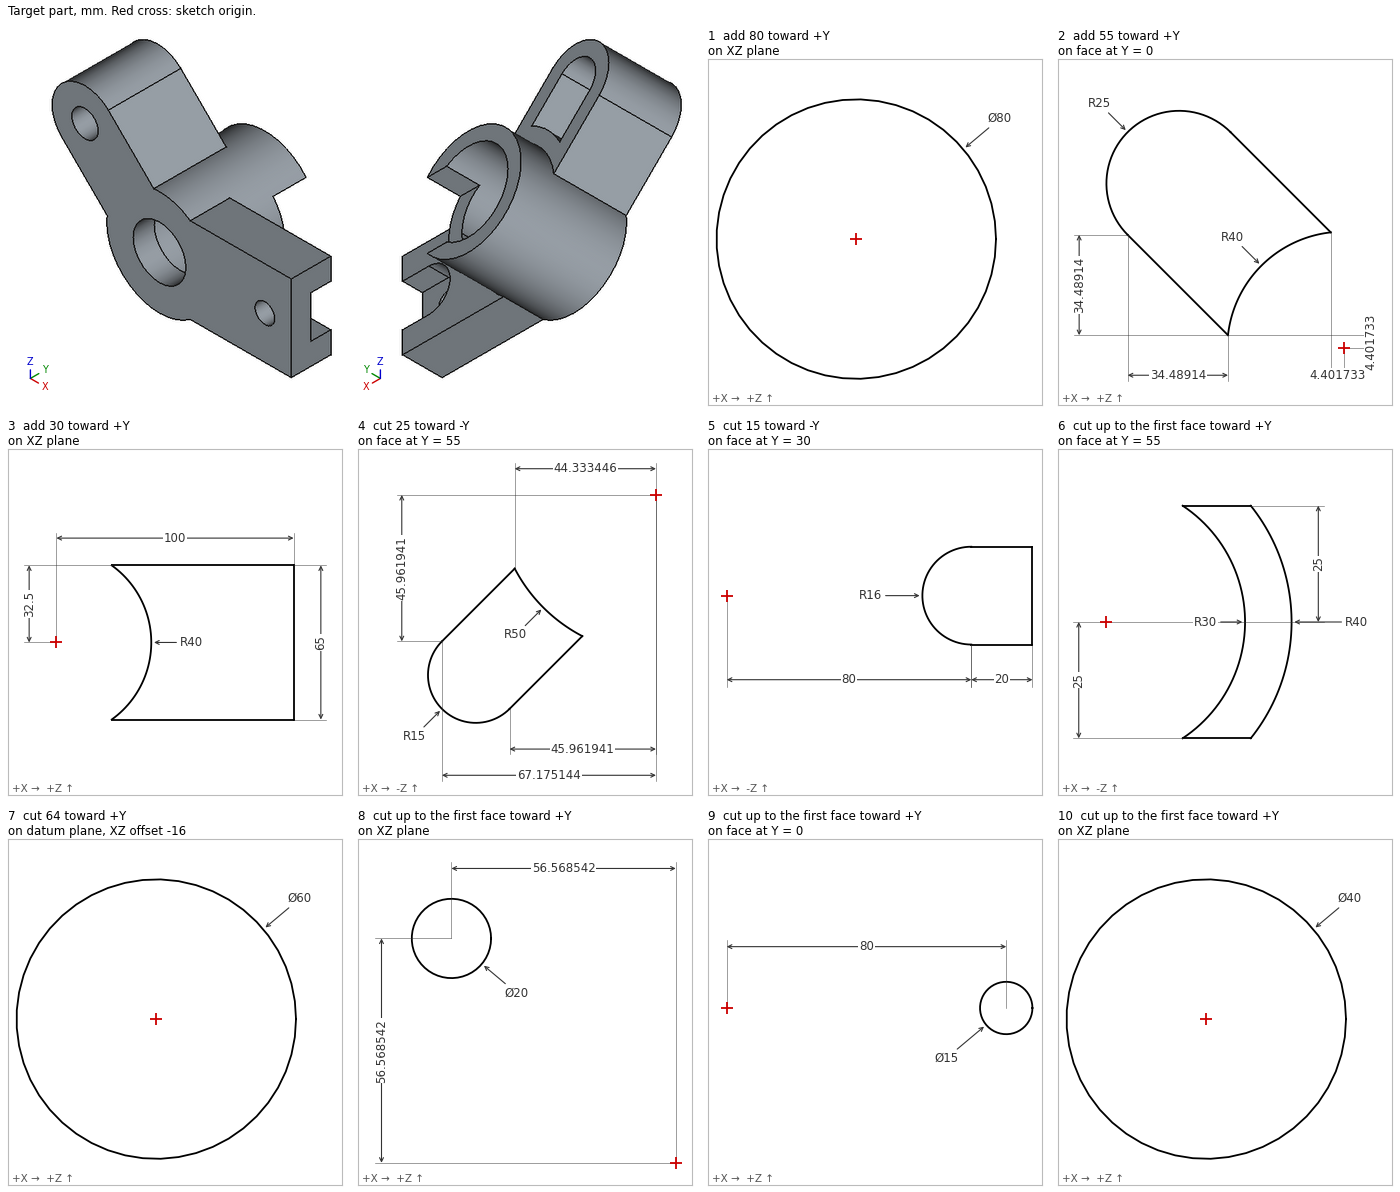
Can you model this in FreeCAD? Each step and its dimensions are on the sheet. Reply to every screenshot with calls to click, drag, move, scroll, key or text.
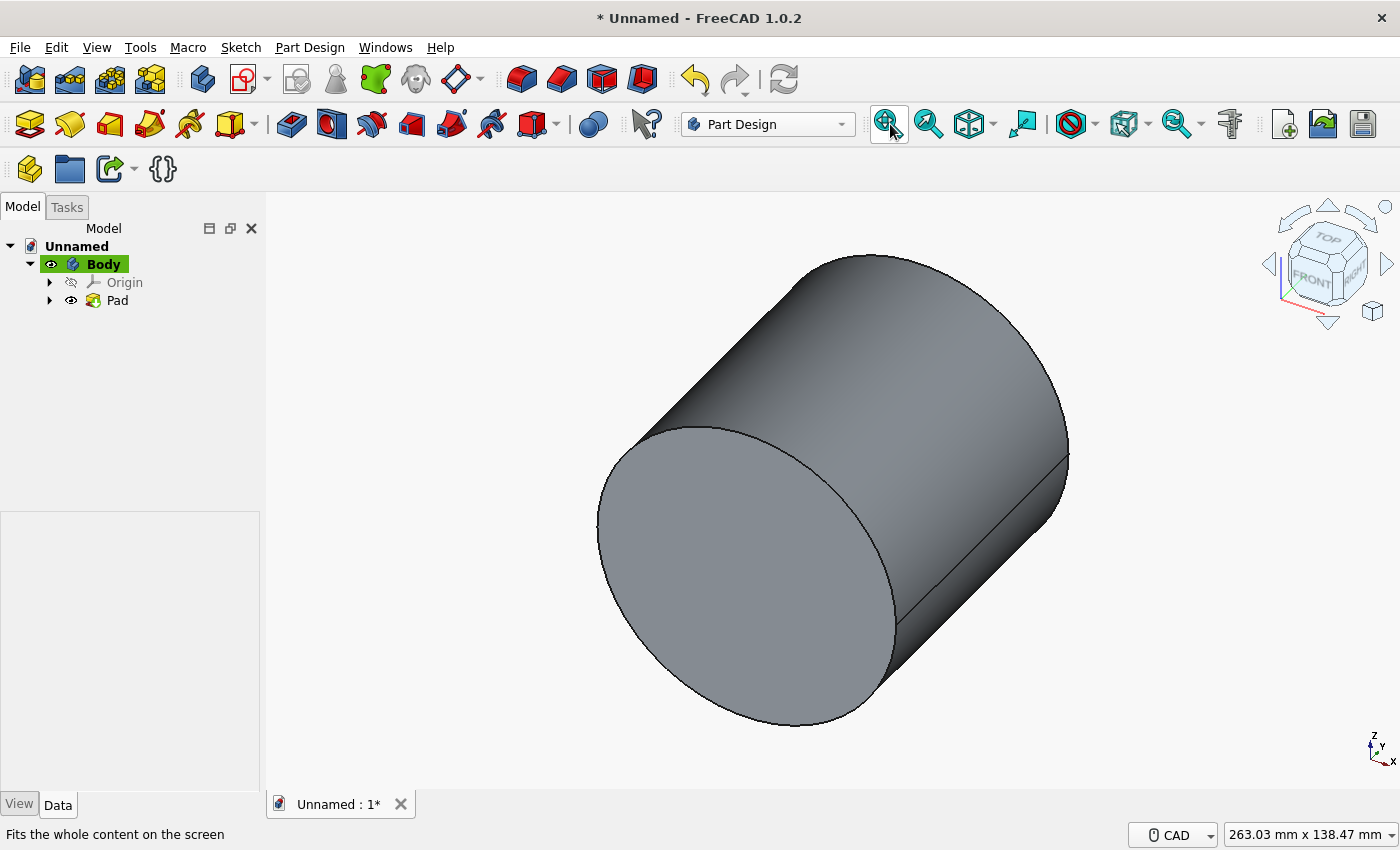
click(747, 575)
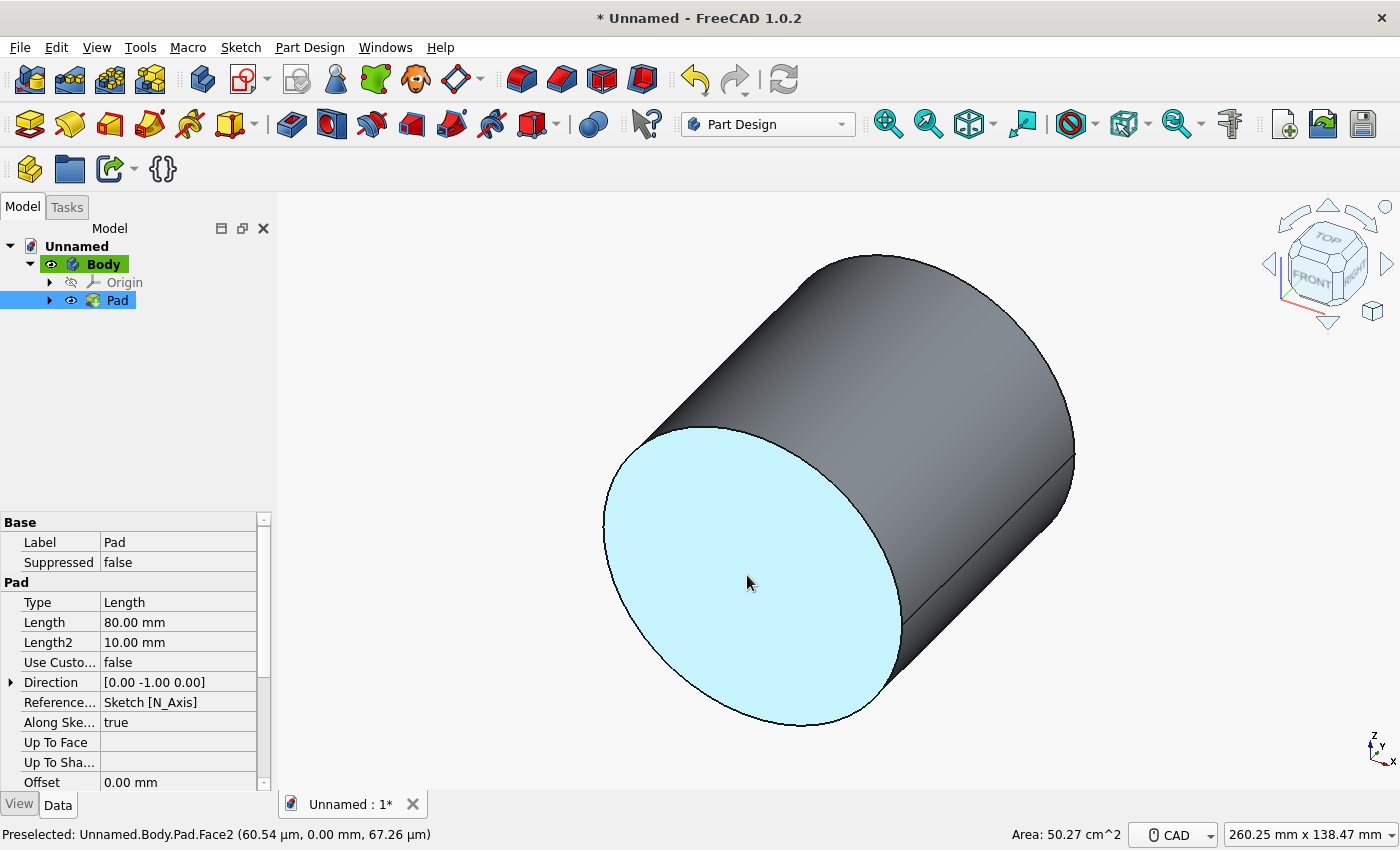
click(244, 80)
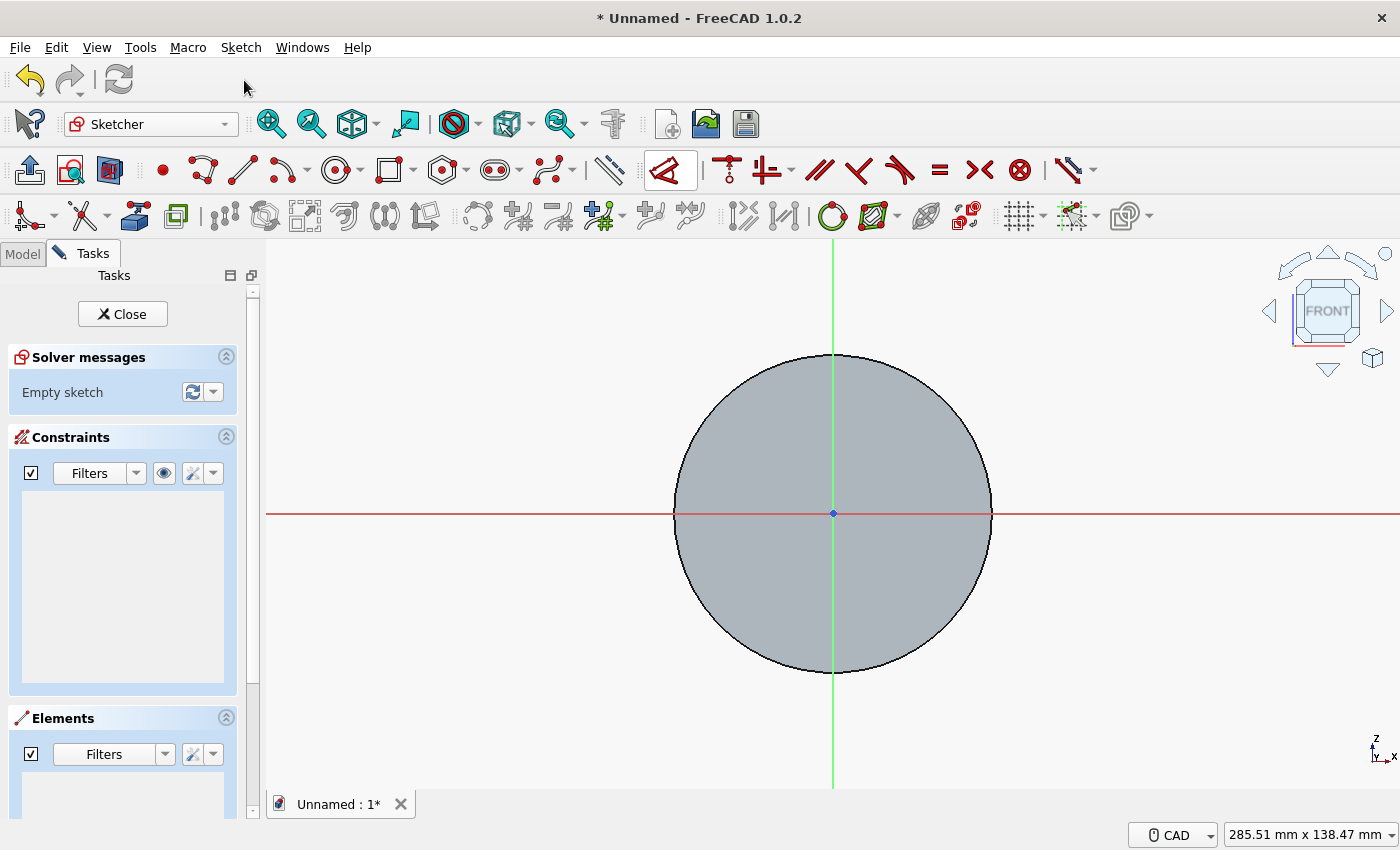
scroll(1121, 761, down, 1)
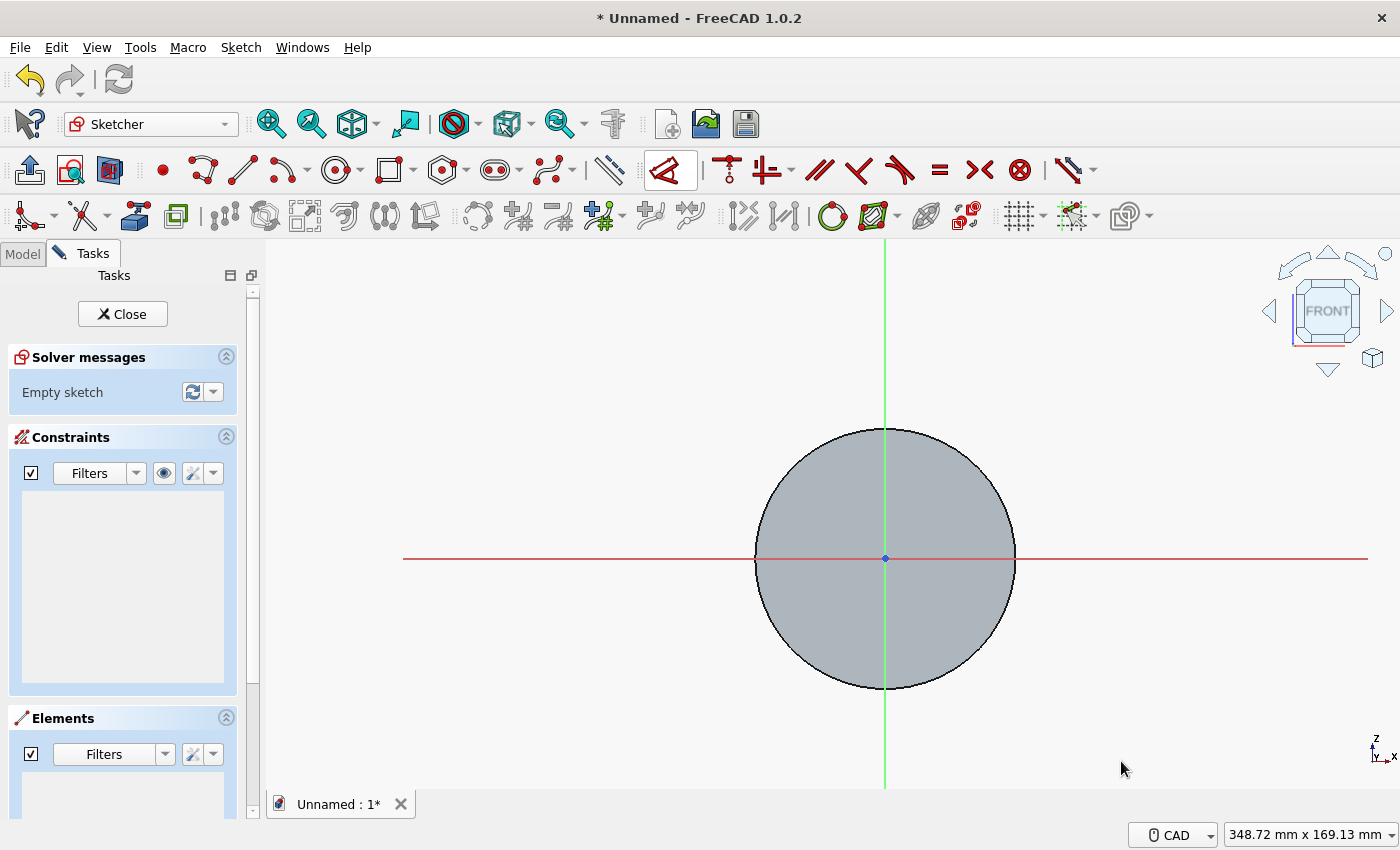
scroll(765, 284, up, 2)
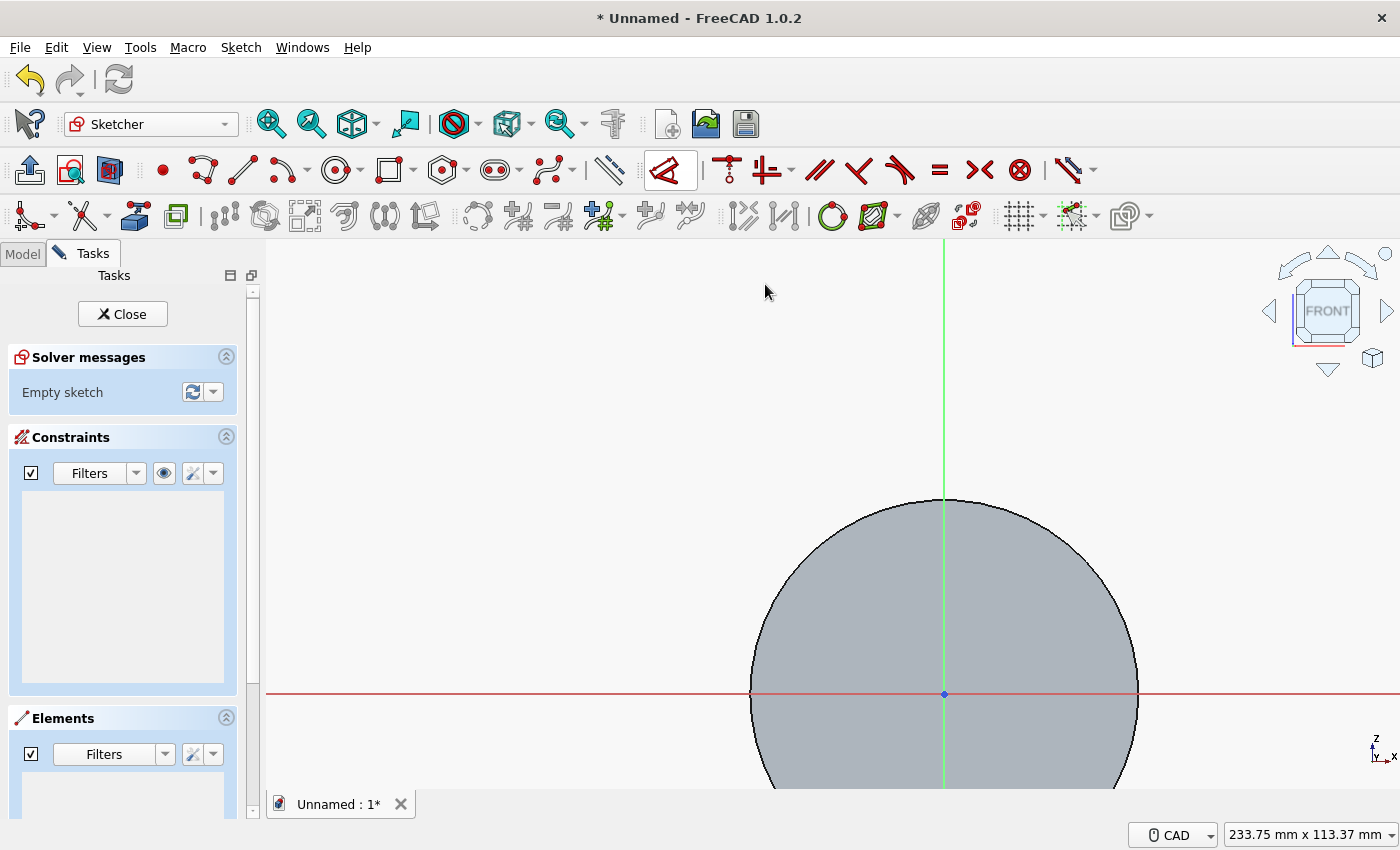
click(244, 170)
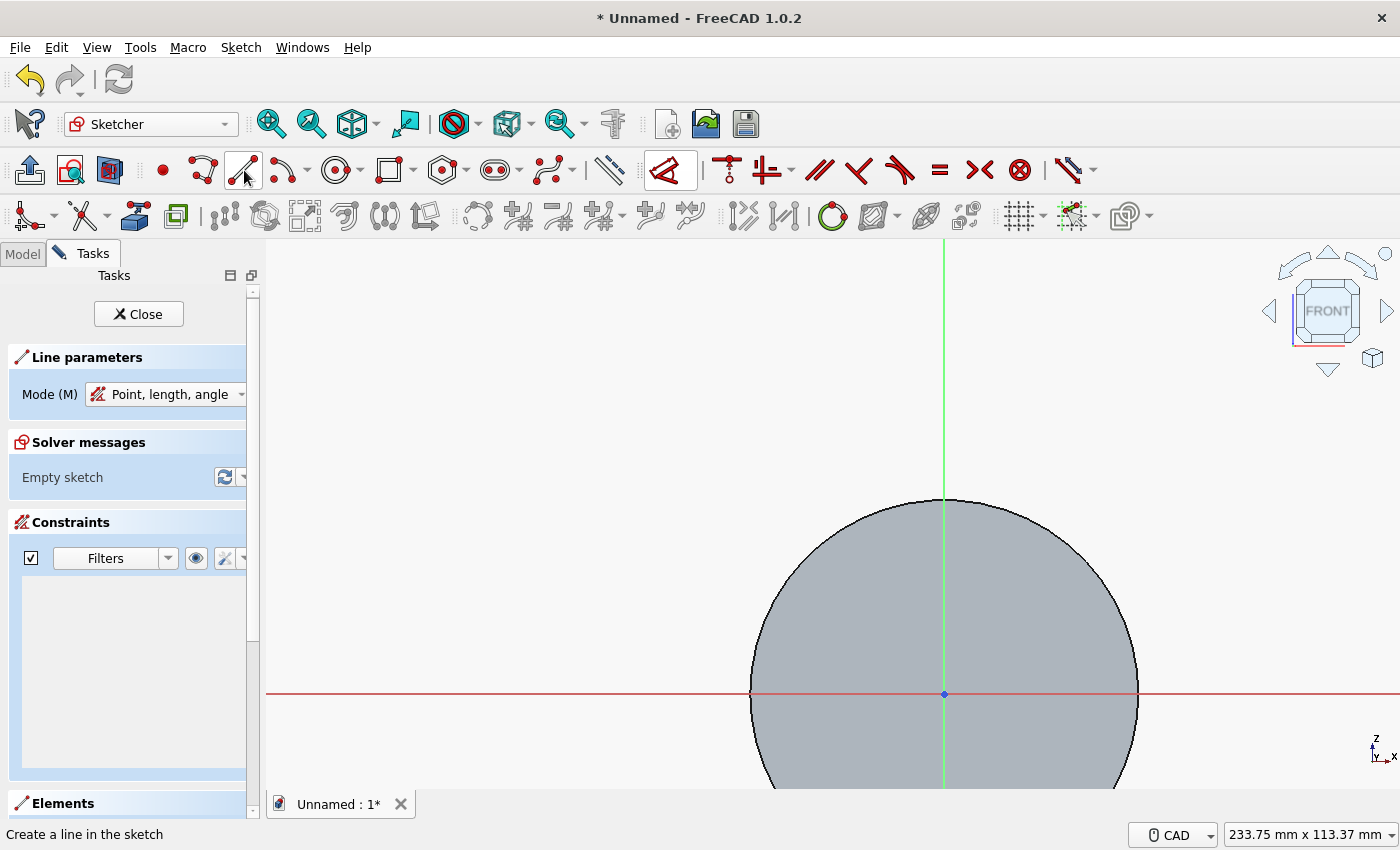
click(751, 673)
click(584, 505)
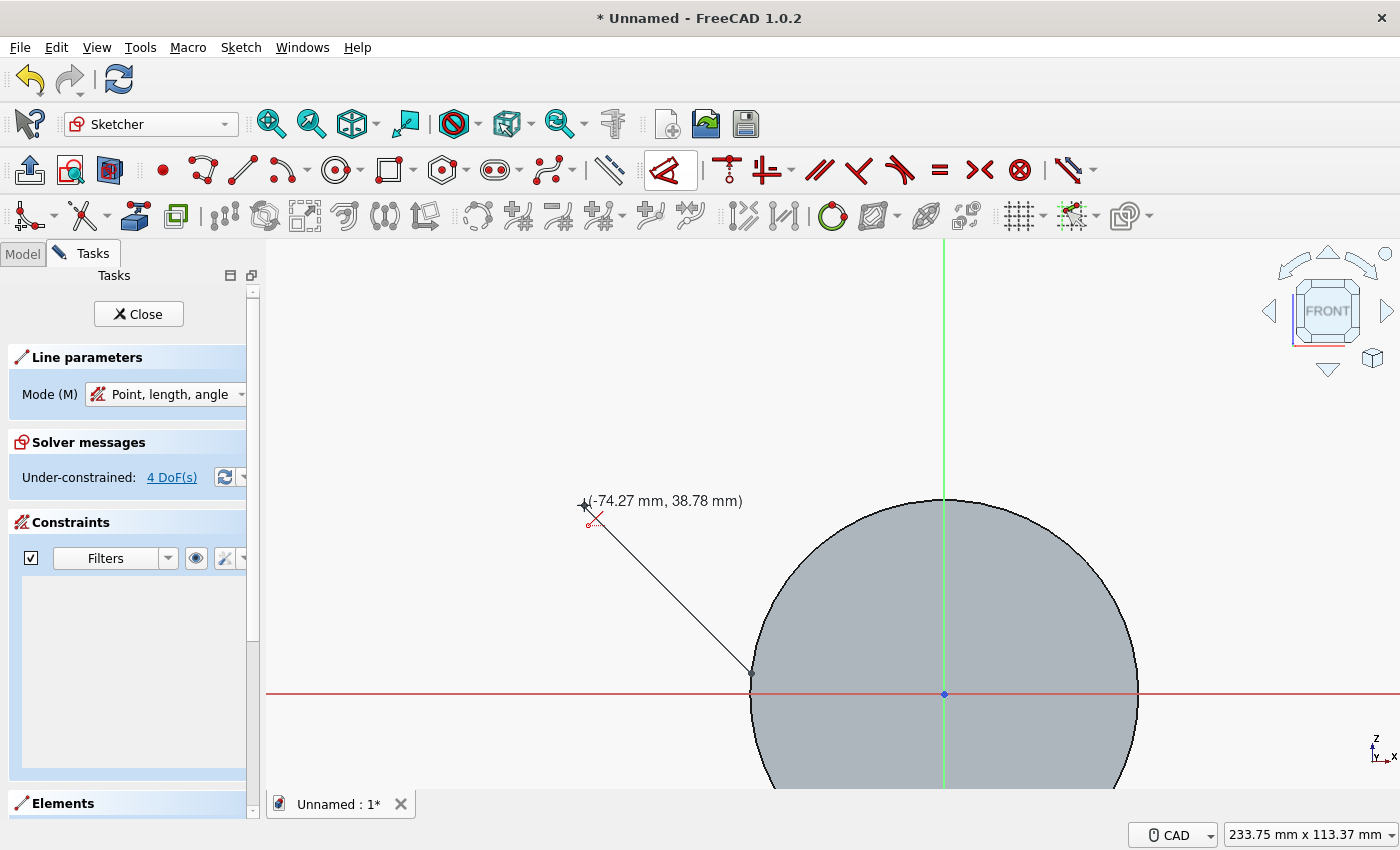
click(756, 334)
click(923, 501)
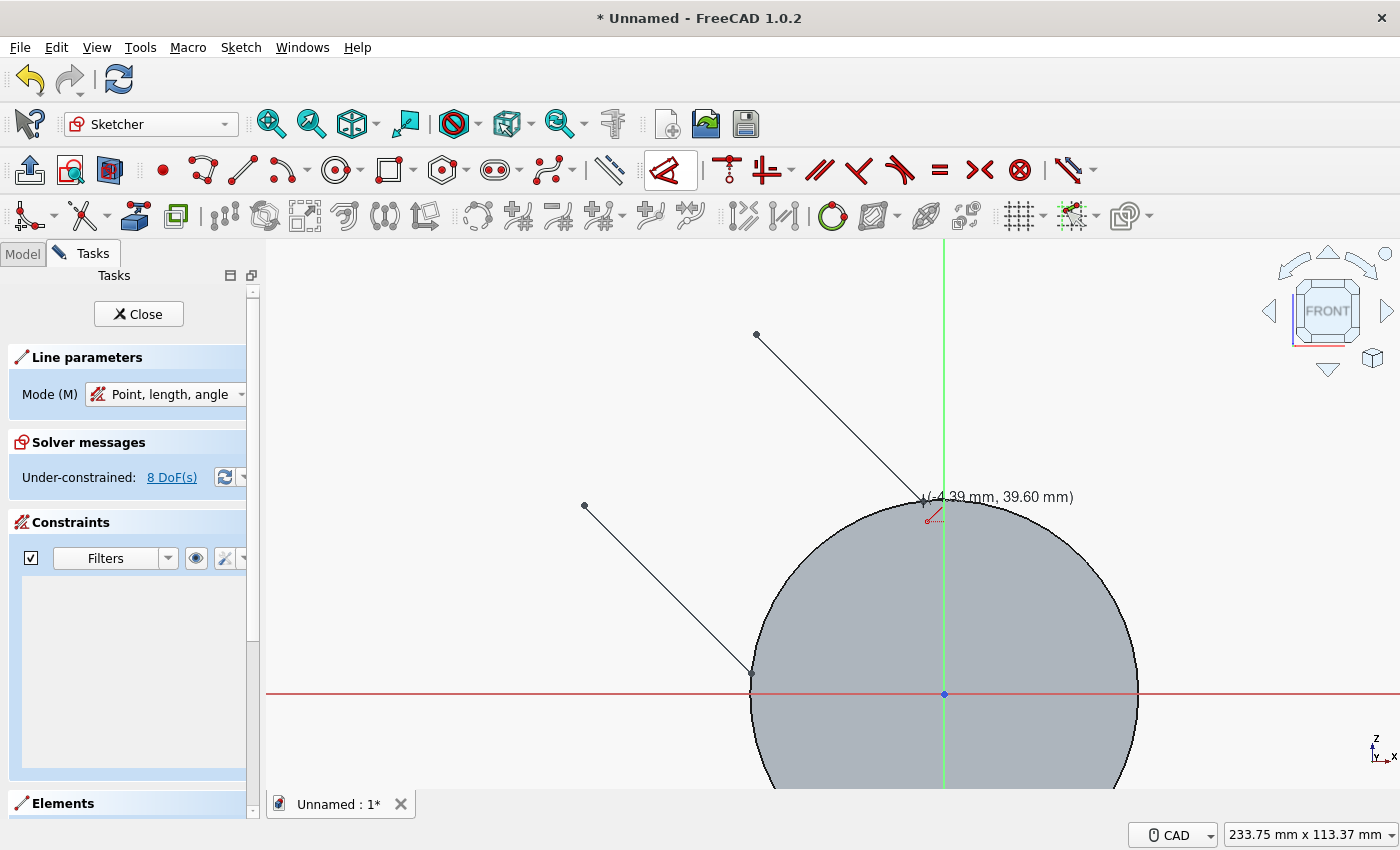
click(310, 170)